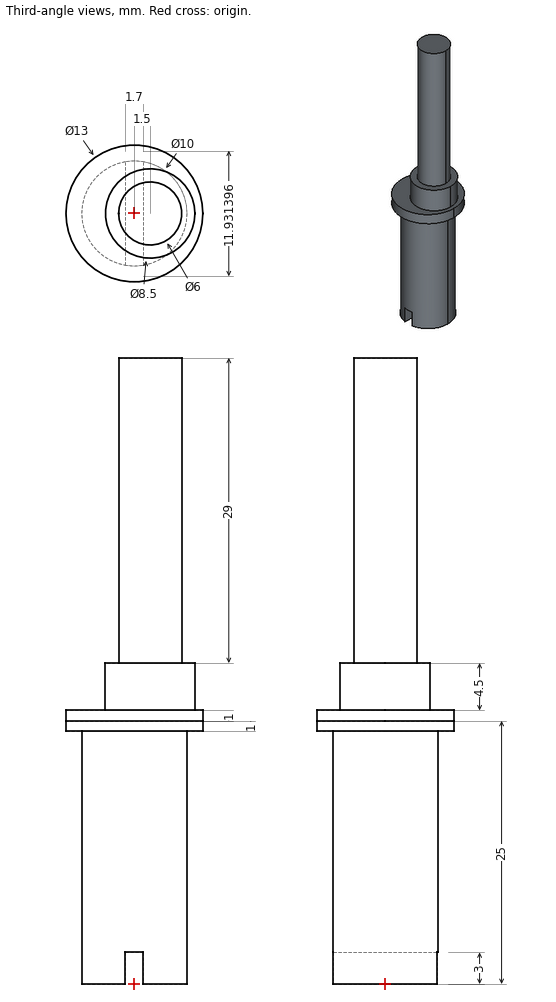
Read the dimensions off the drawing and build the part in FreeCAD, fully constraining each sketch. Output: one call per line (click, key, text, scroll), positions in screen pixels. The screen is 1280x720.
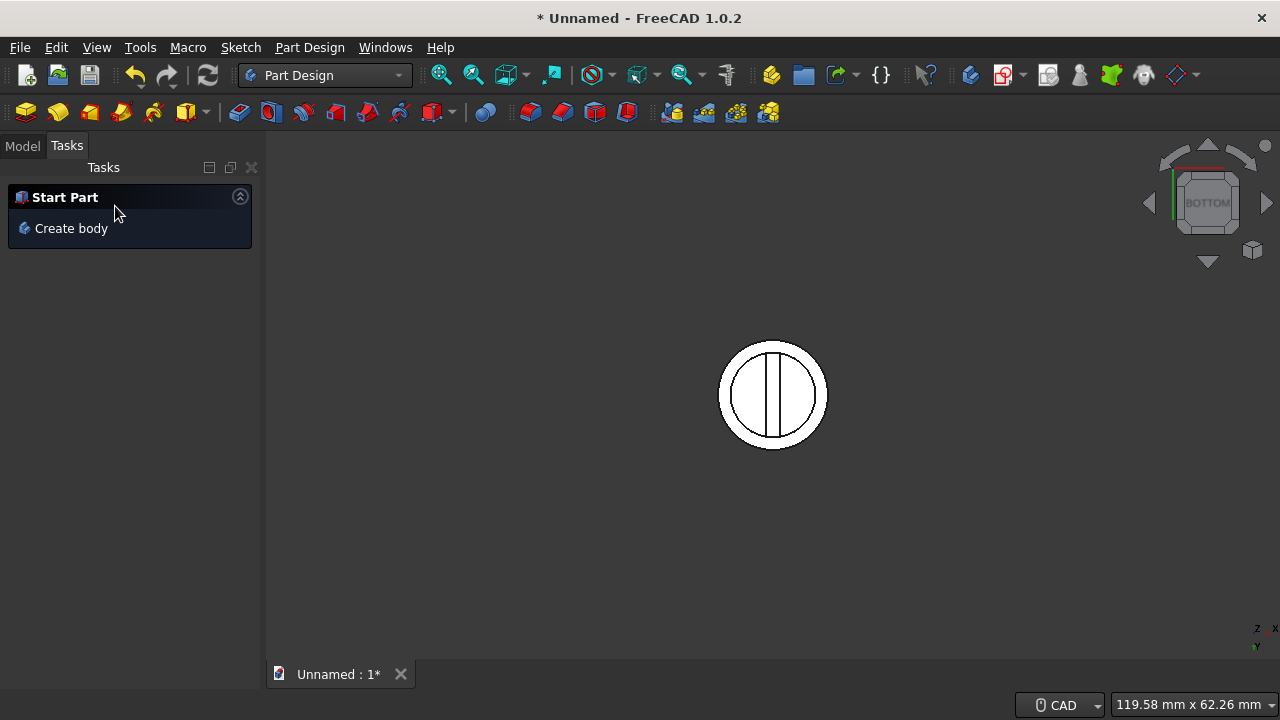
click(442, 76)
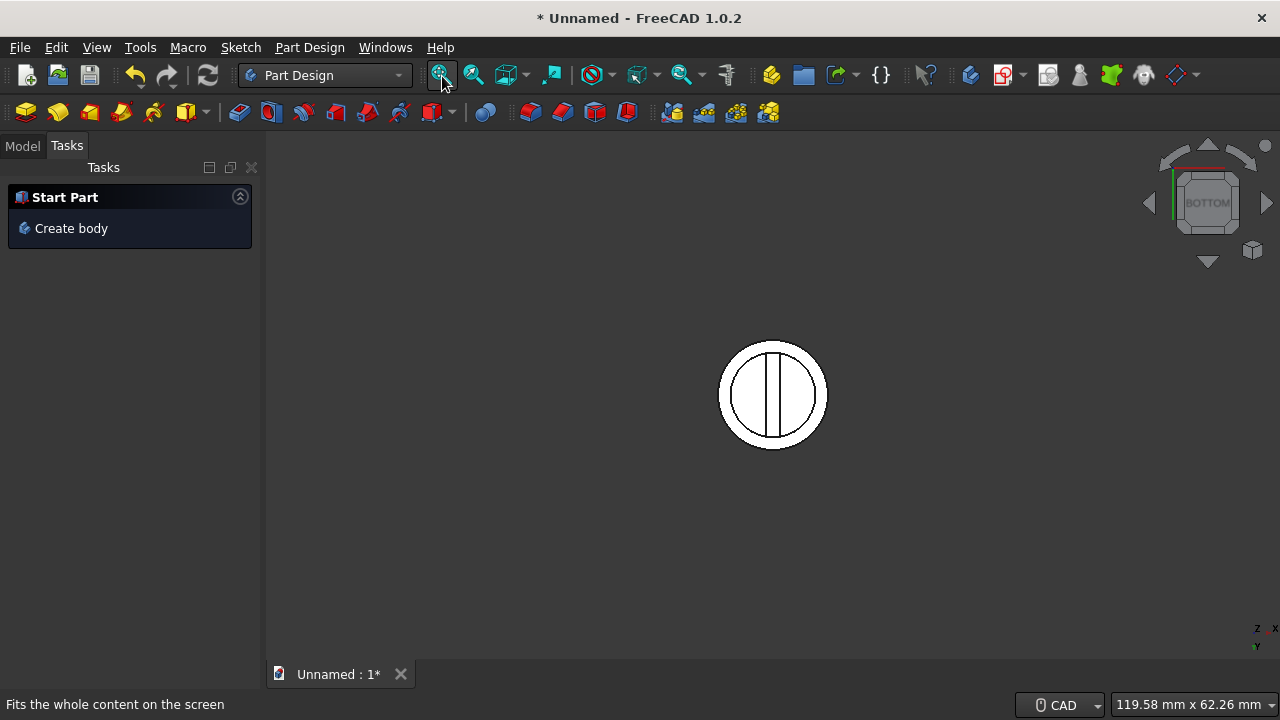
click(23, 145)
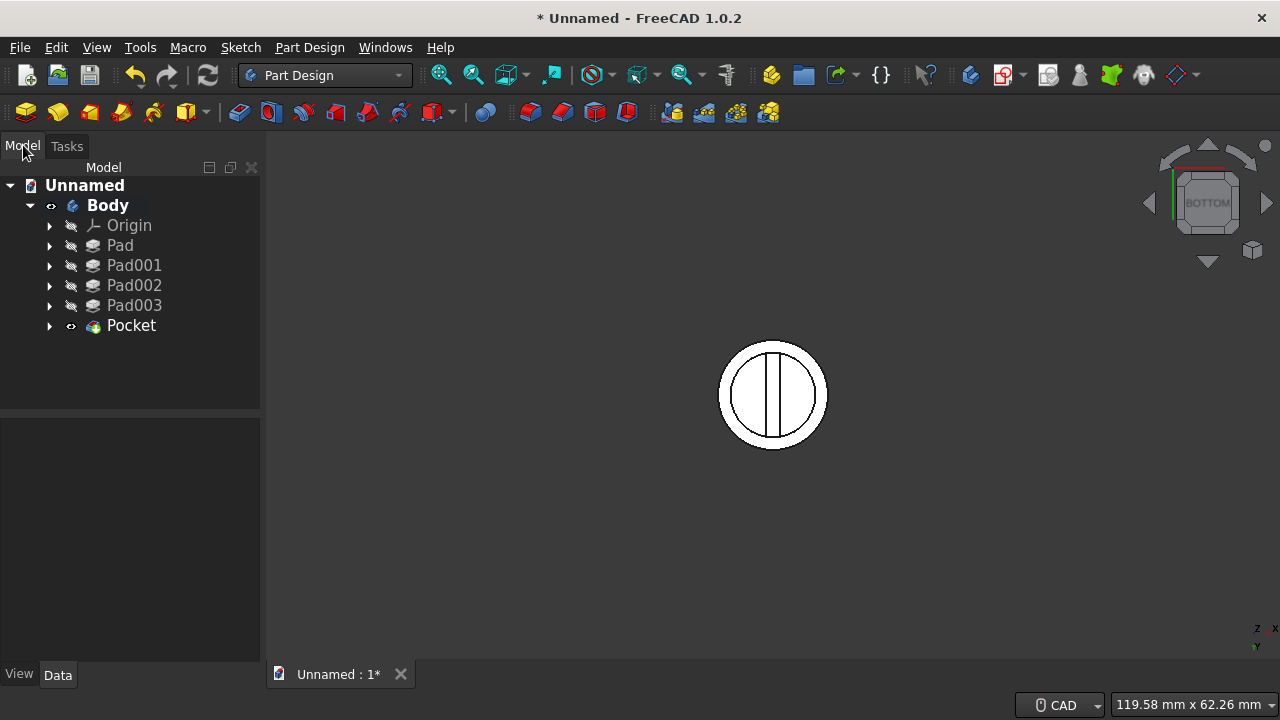
click(50, 226)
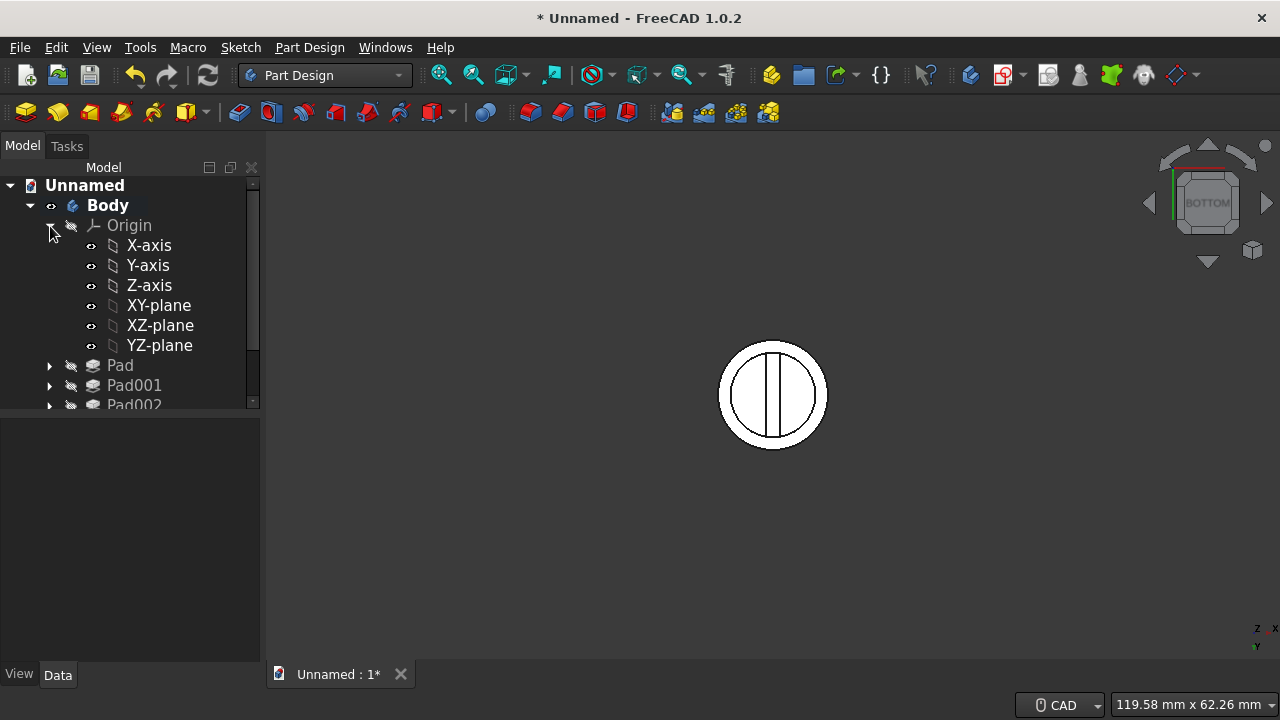
click(136, 306)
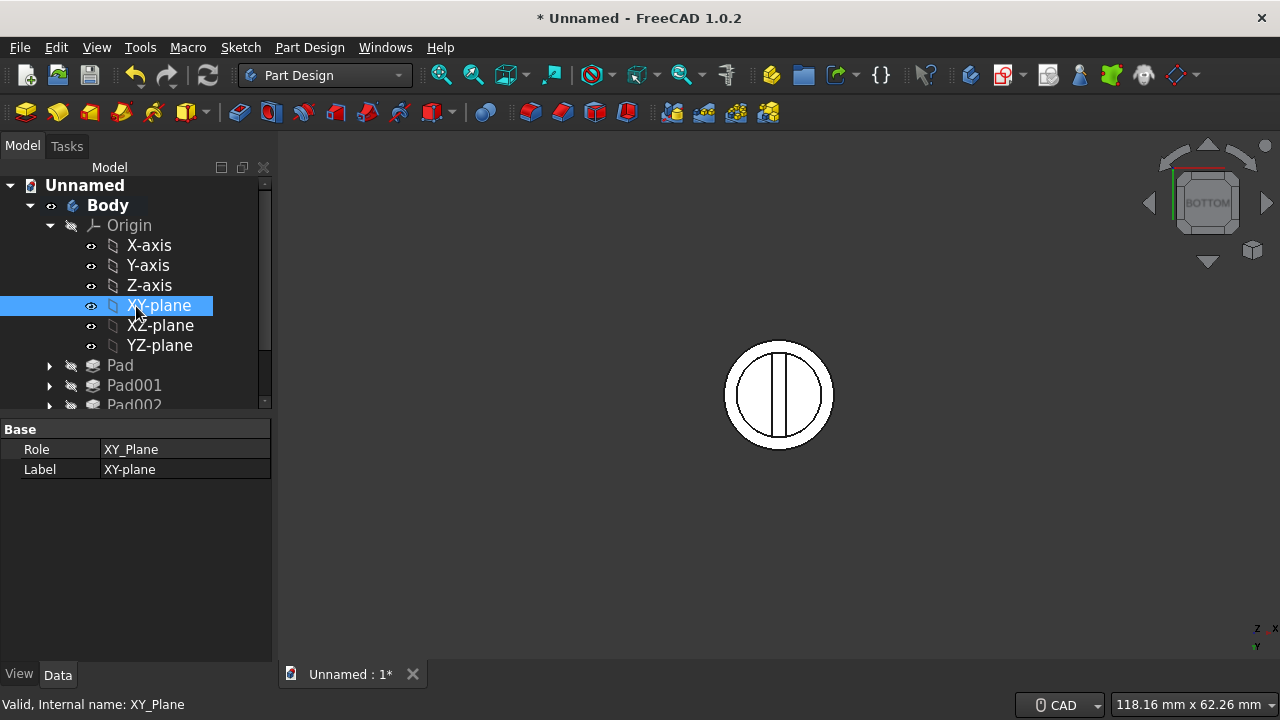
click(1176, 76)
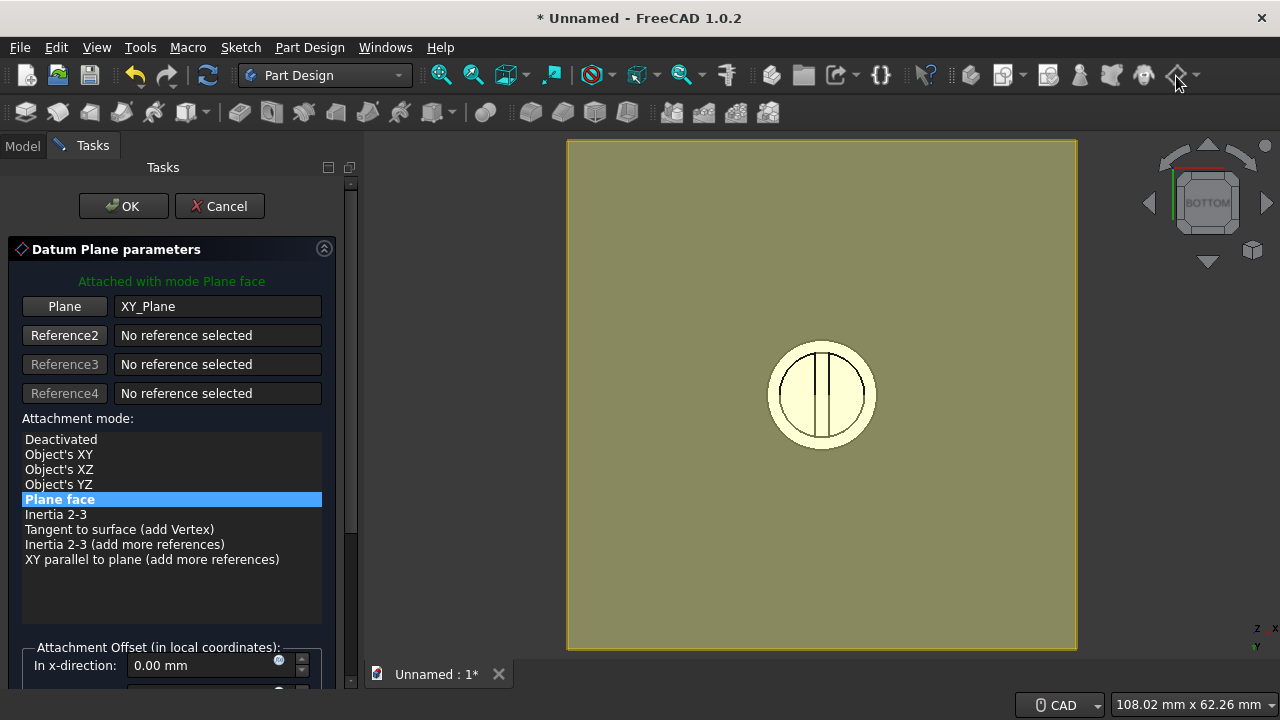
scroll(351, 432, down, 2)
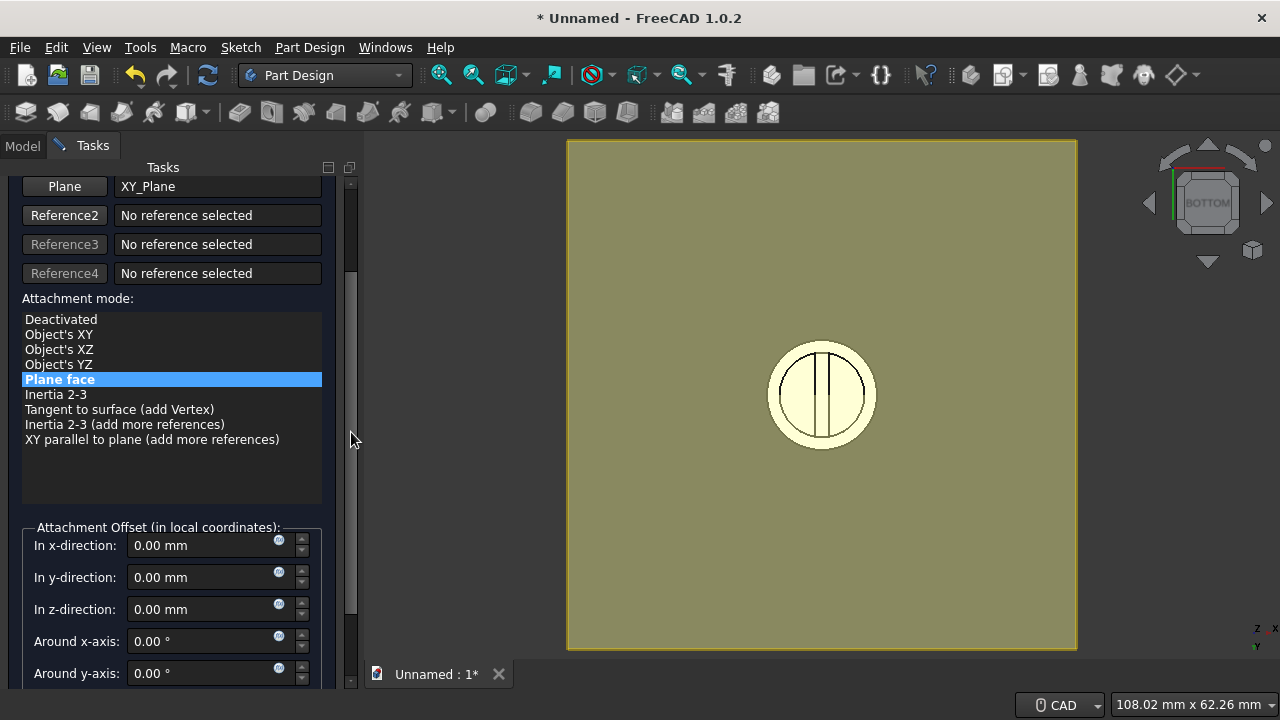
triple_click(210, 609)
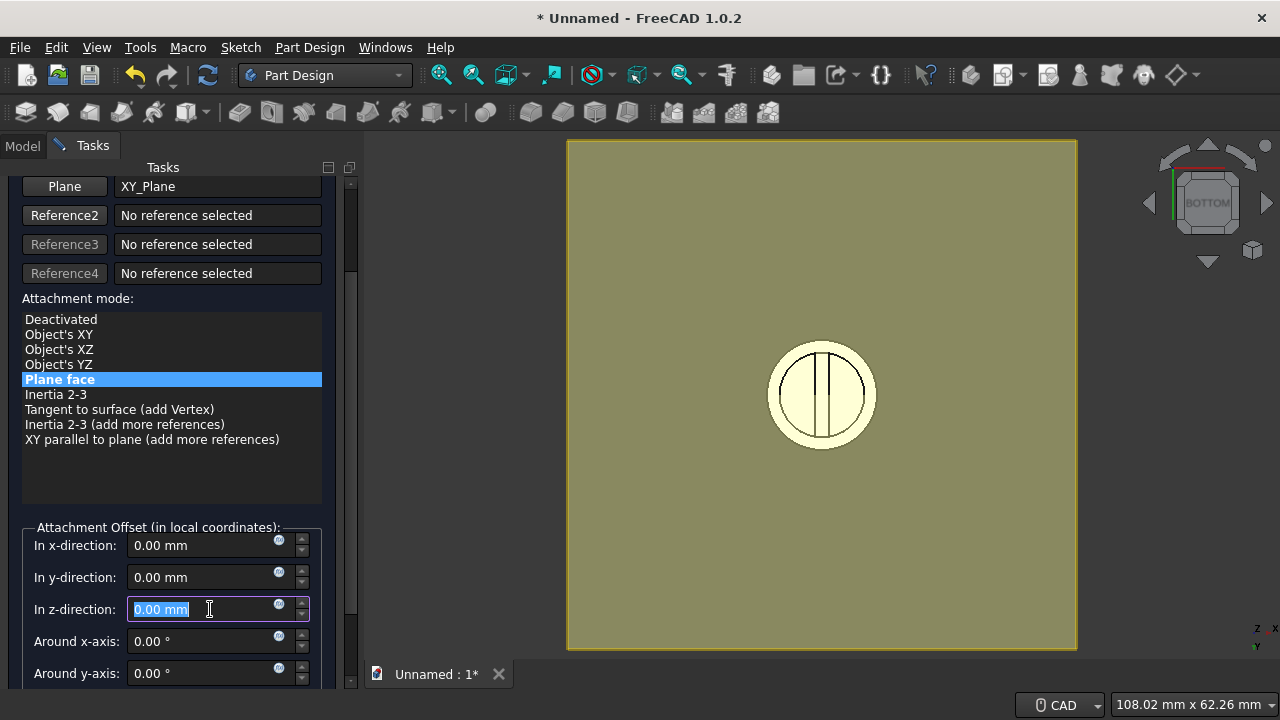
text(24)
key(Tab)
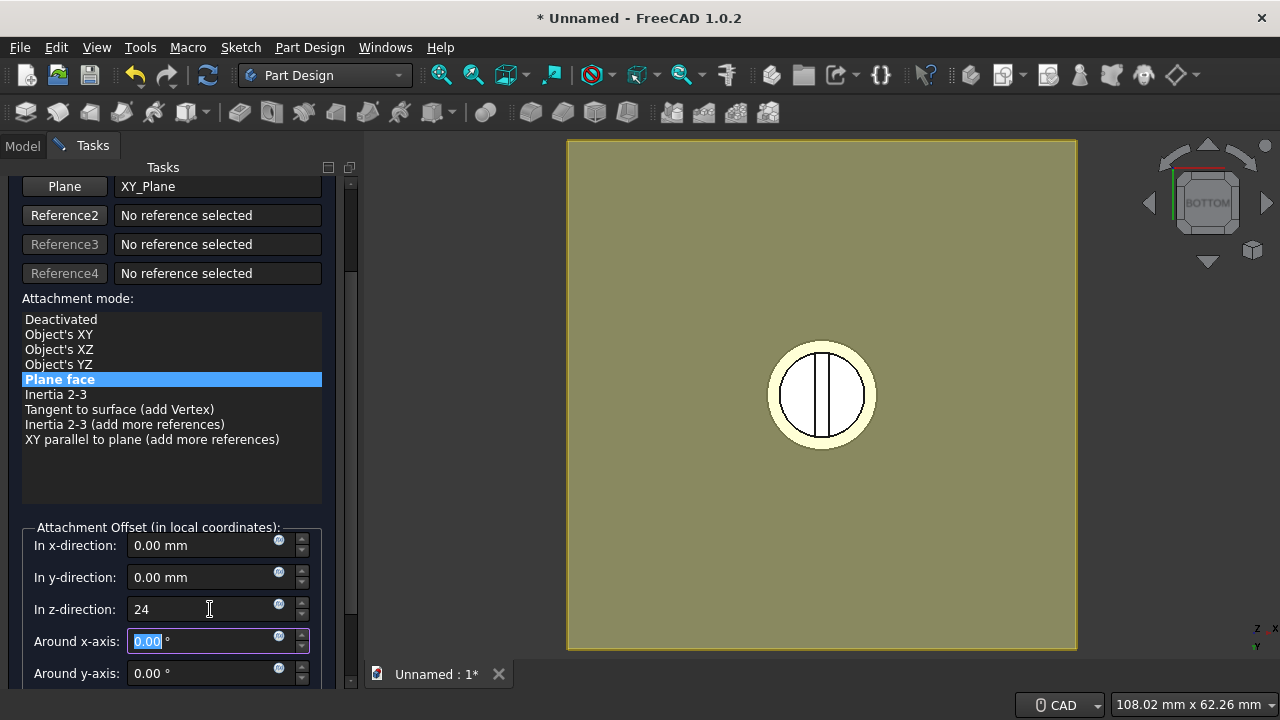
scroll(351, 432, up, 3)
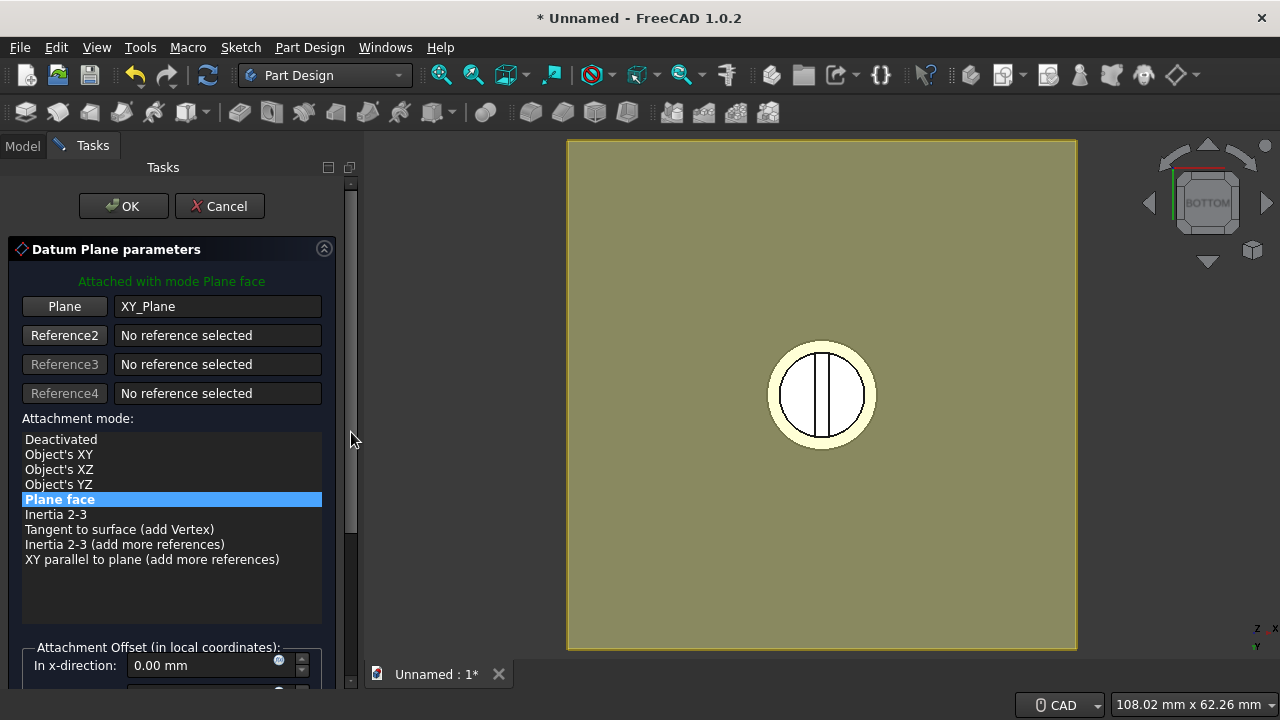
click(124, 206)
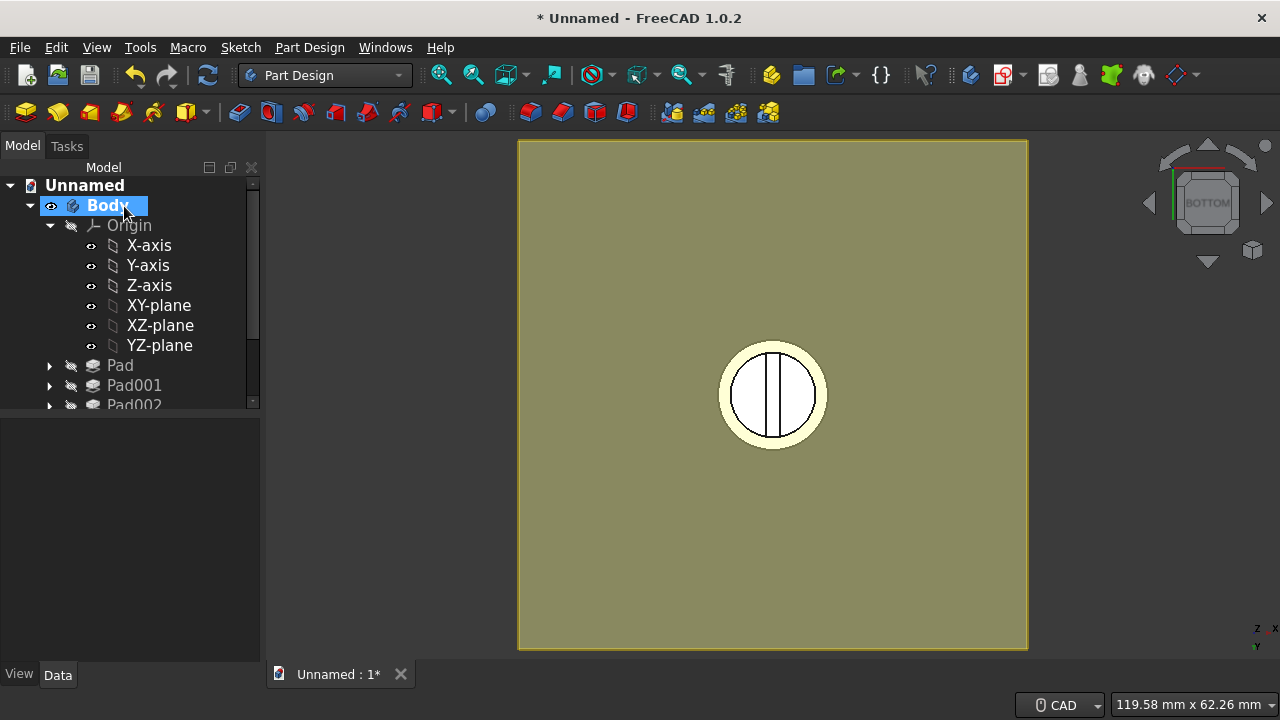
scroll(100, 301, down, 3)